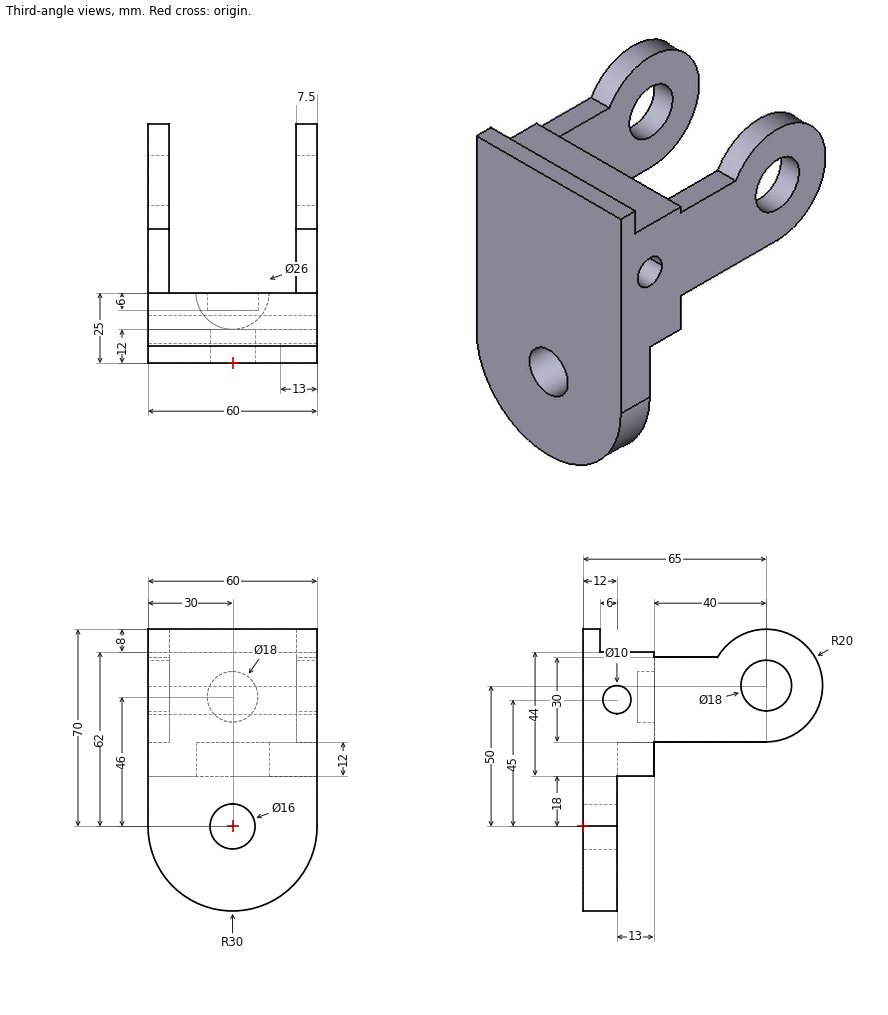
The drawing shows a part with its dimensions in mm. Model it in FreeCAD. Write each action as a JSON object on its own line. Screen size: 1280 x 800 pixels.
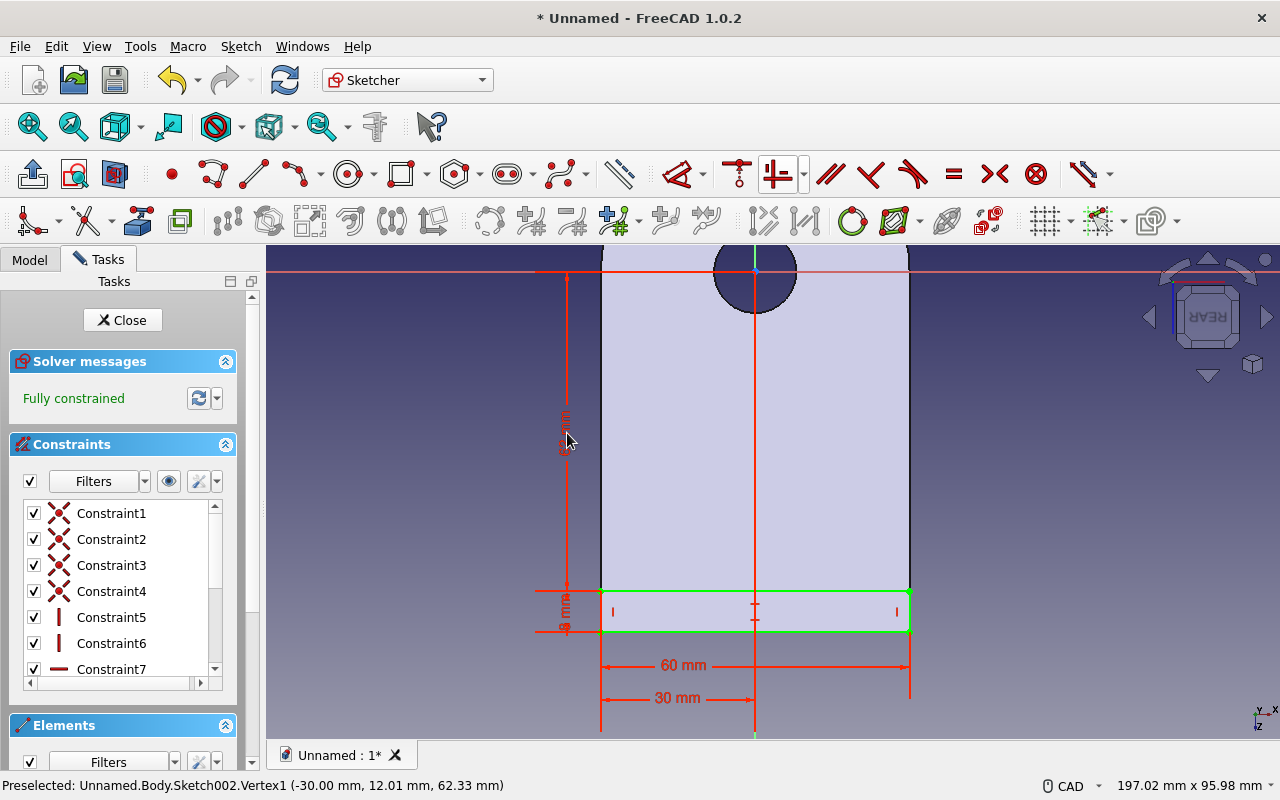
{"action": "left_click", "coordinate": [123, 320]}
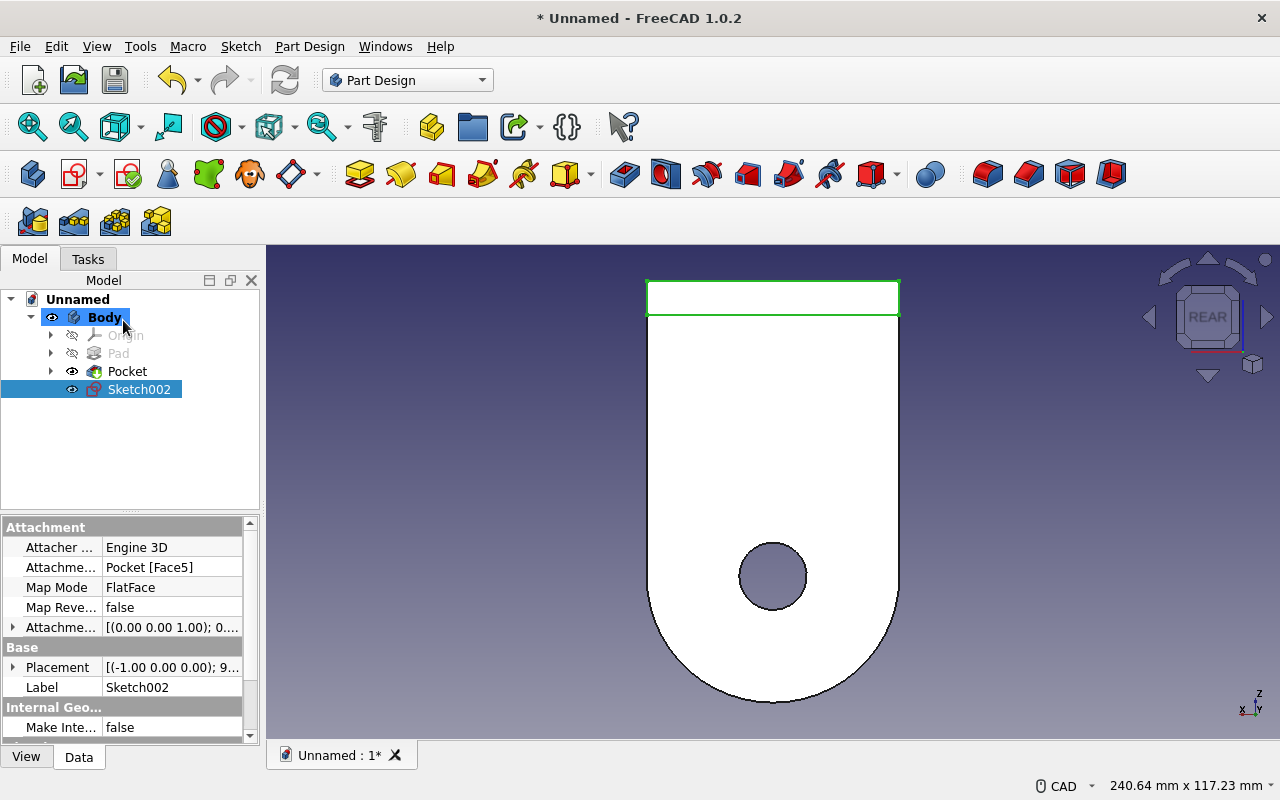
{"action": "left_click", "coordinate": [625, 174]}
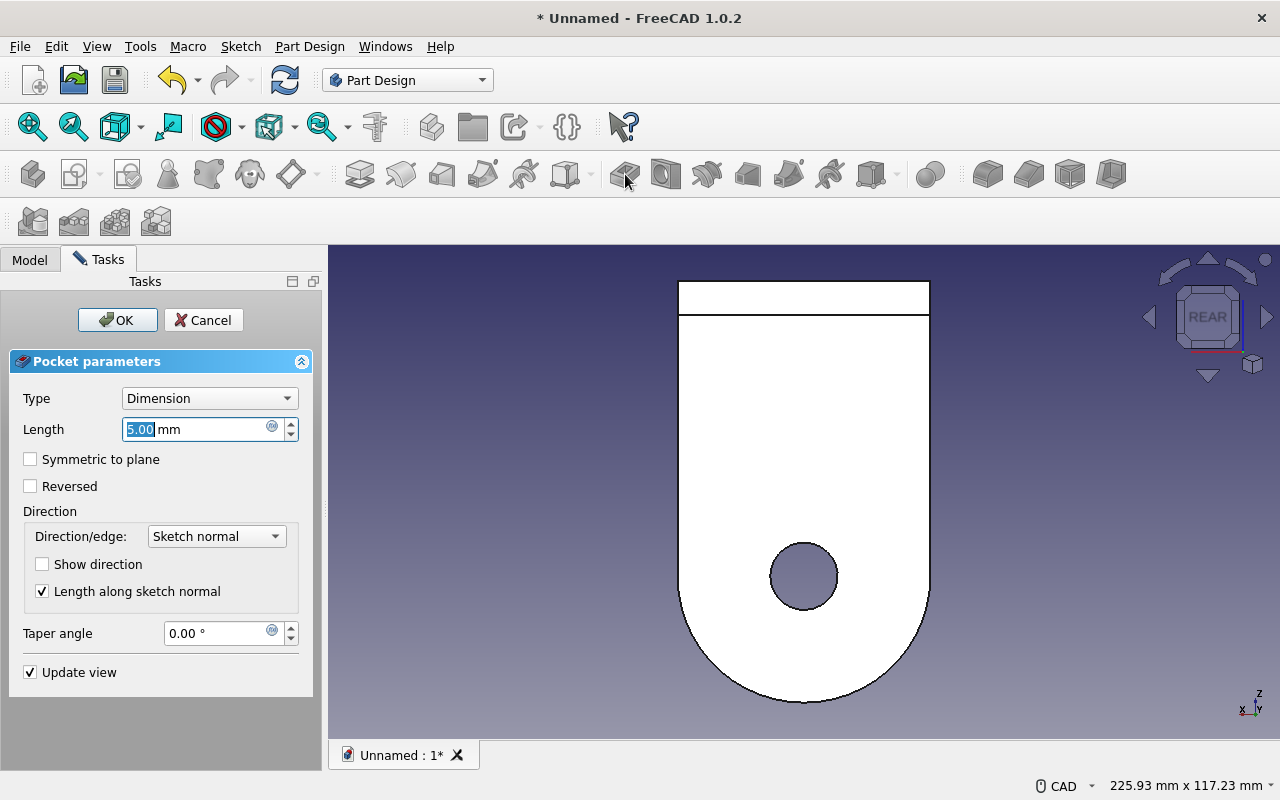
{"action": "type", "text": "6"}
{"action": "key", "text": "Tab"}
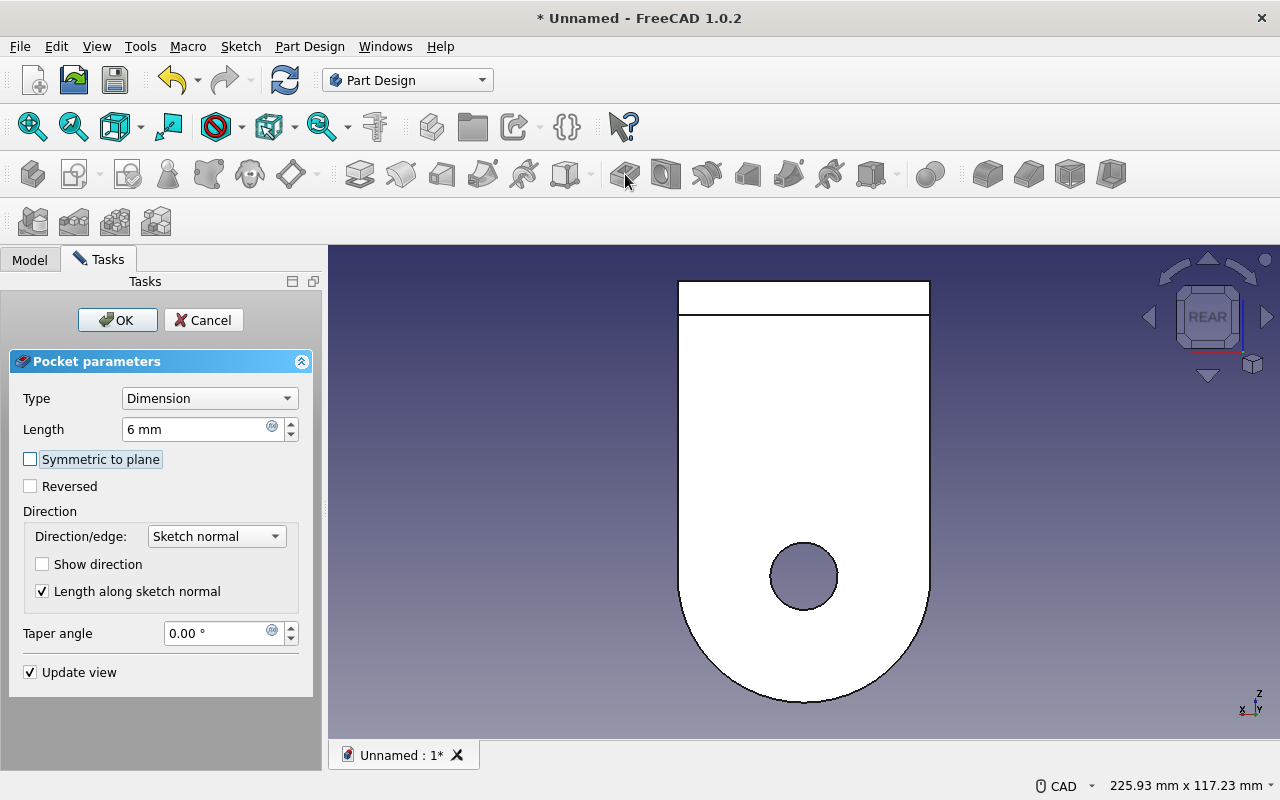
{"action": "left_click", "coordinate": [118, 320]}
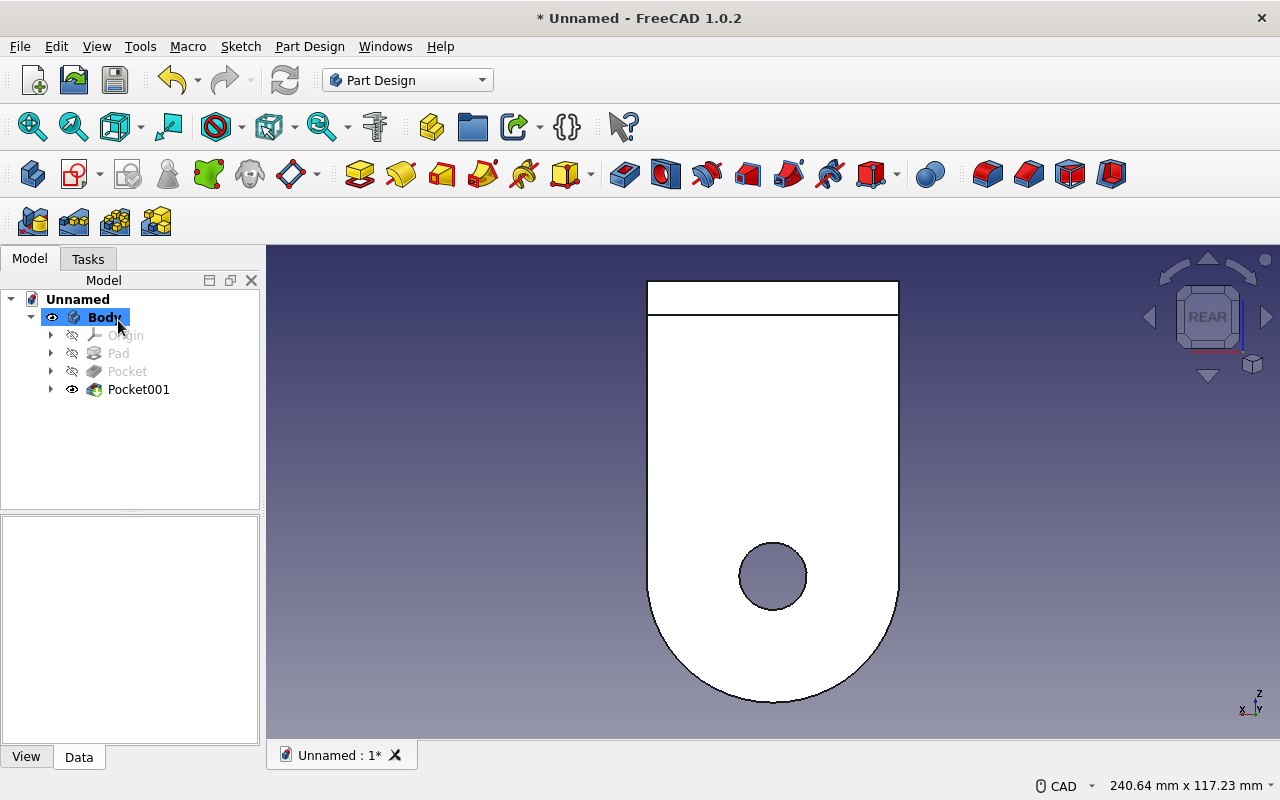
{"action": "key", "text": "0"}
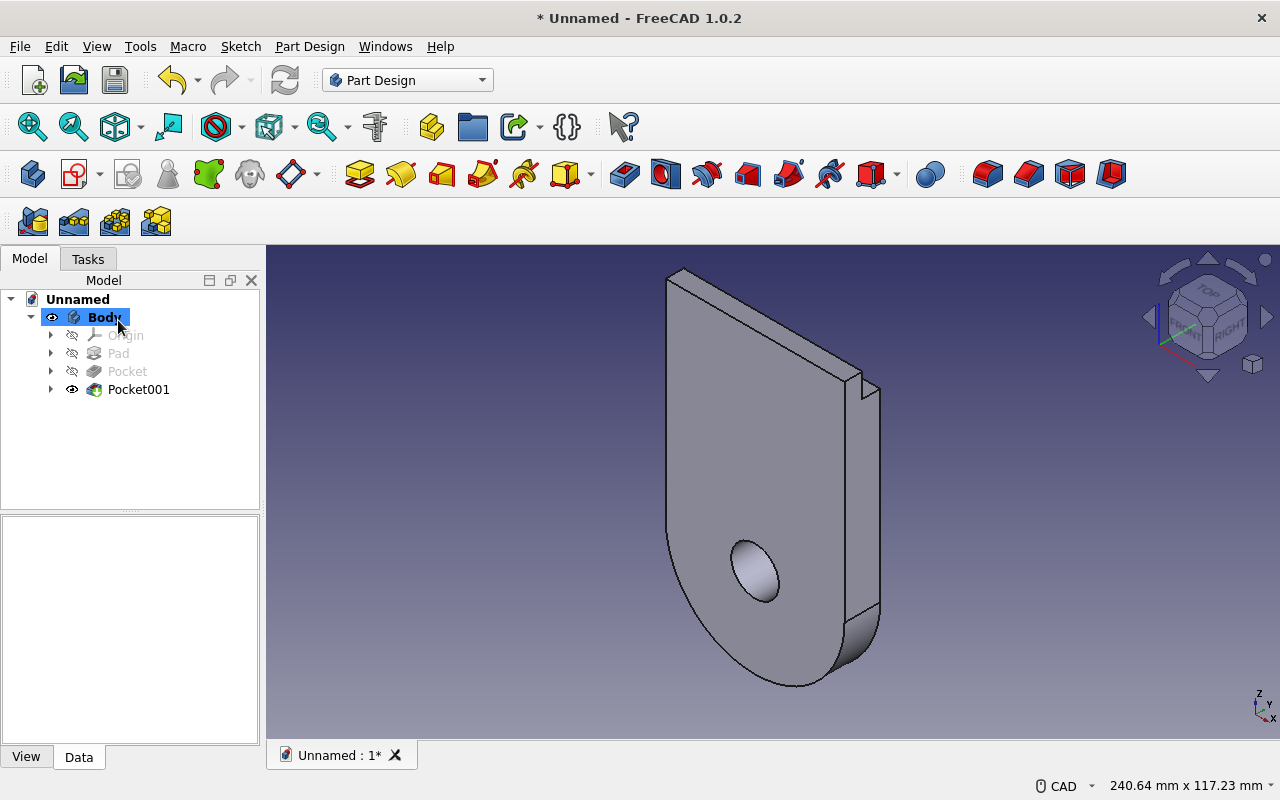
{"action": "left_click", "coordinate": [862, 422]}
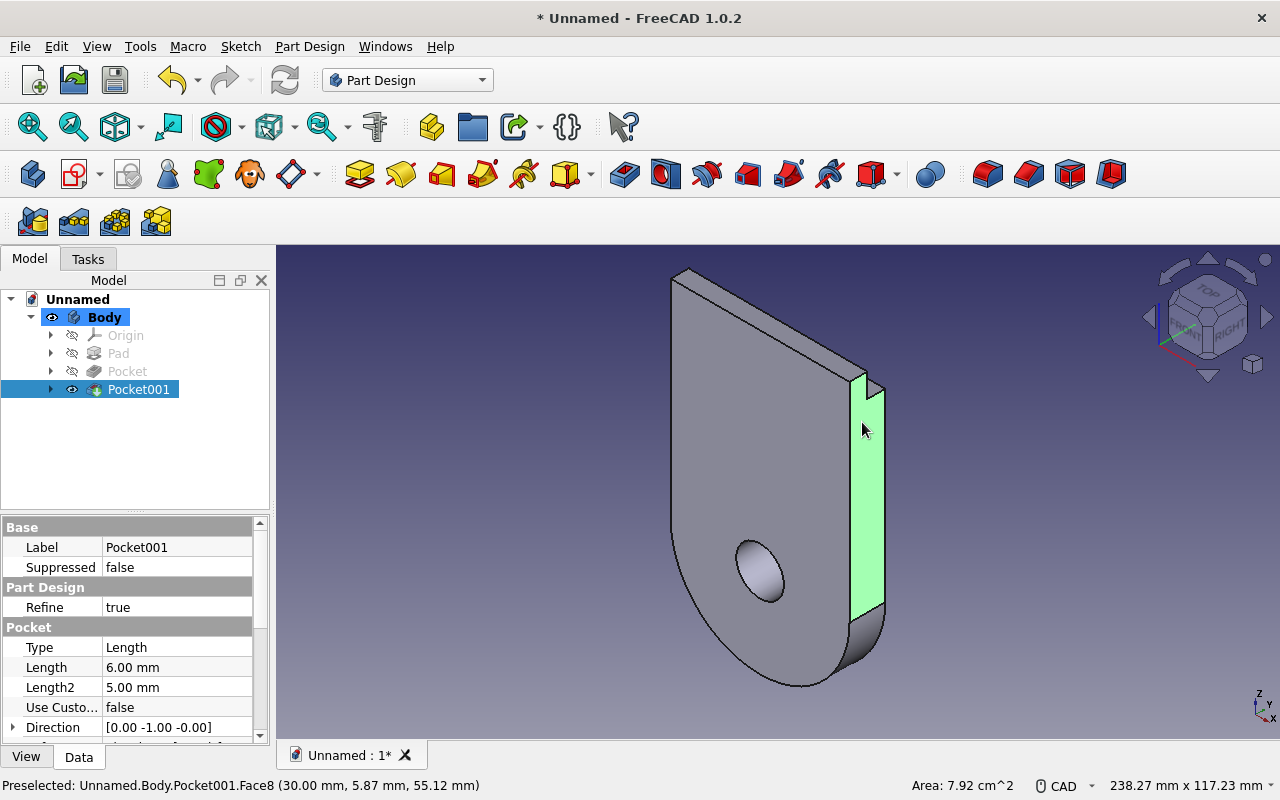
{"action": "left_click", "coordinate": [74, 174]}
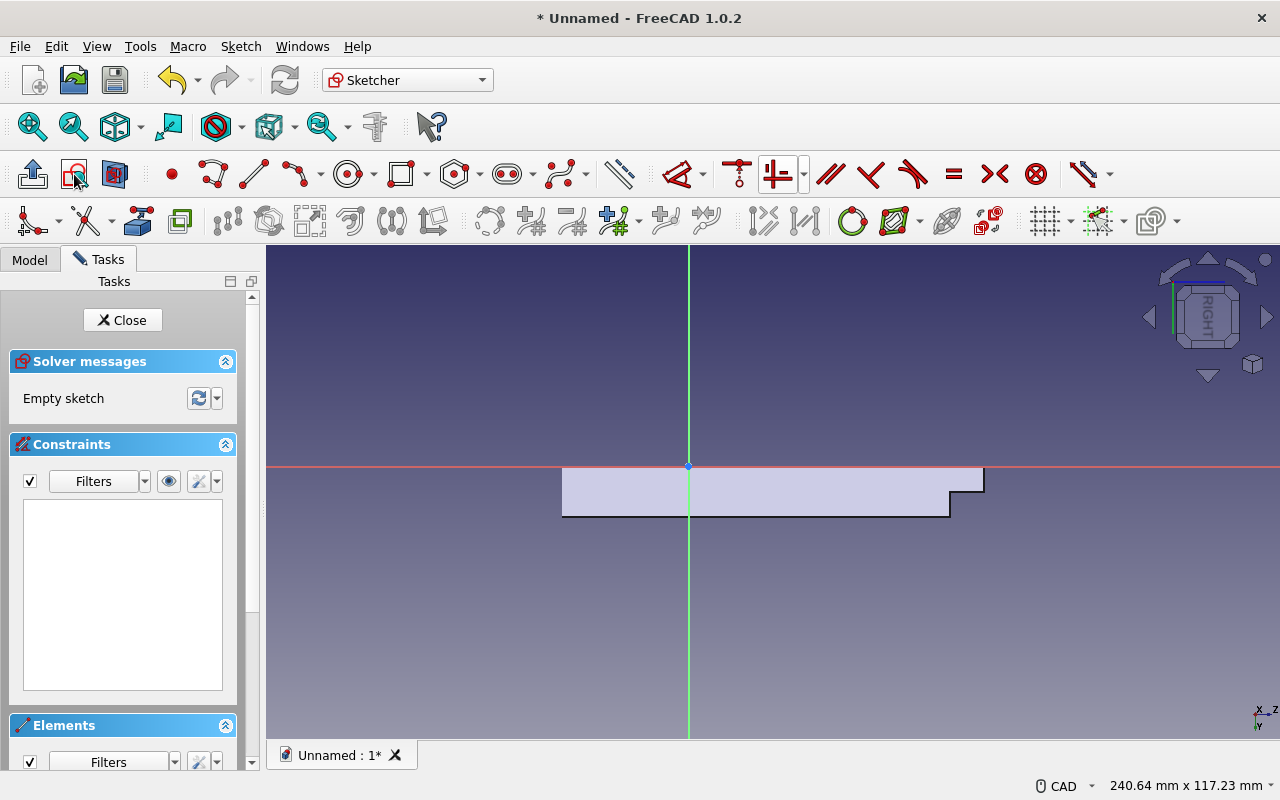
{"action": "scroll", "coordinate": [913, 542], "scroll_direction": "up", "scroll_amount": 4}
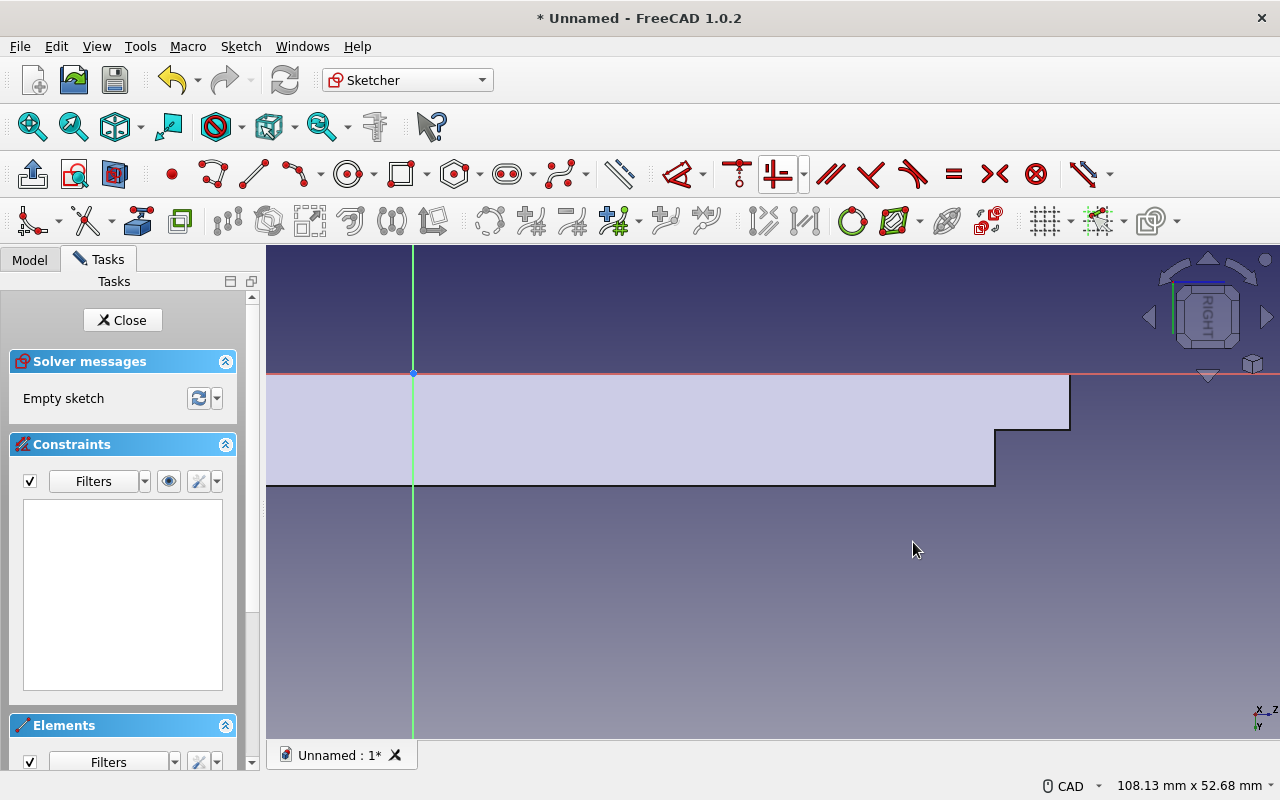
{"action": "key", "text": "g r"}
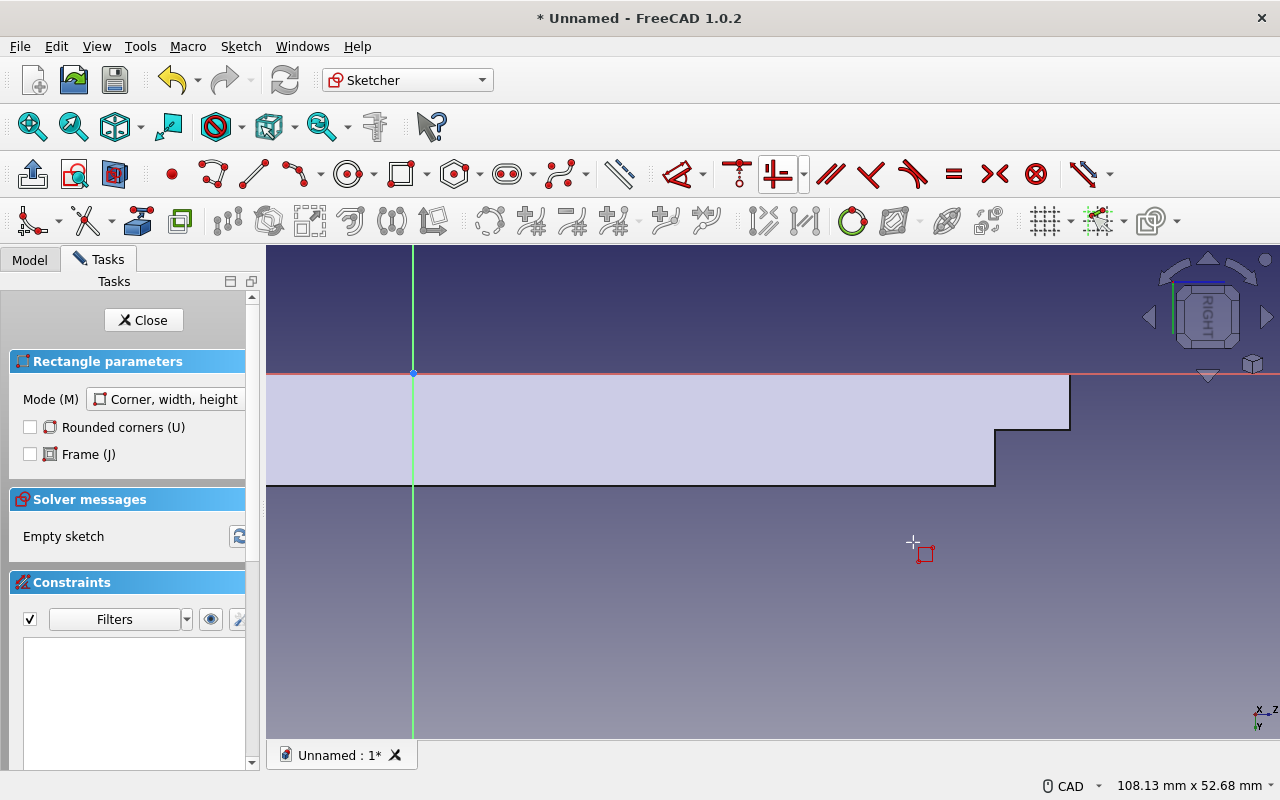
{"action": "left_click", "coordinate": [582, 486]}
{"action": "left_click", "coordinate": [995, 608]}
{"action": "key", "text": "Escape"}